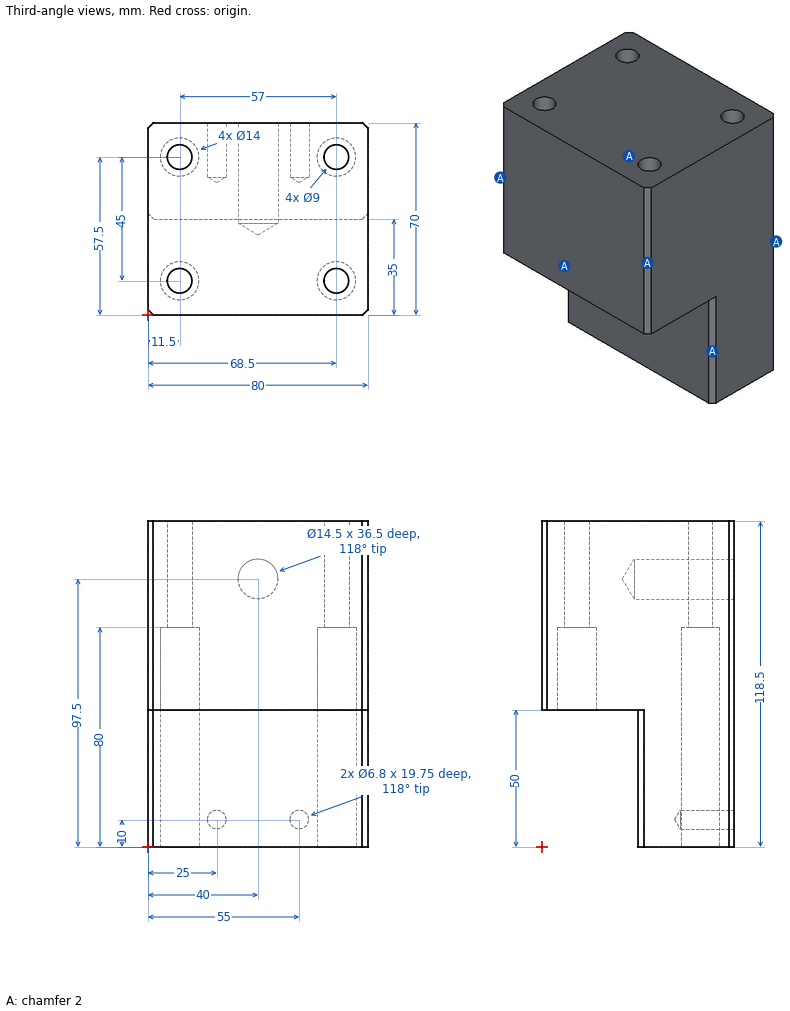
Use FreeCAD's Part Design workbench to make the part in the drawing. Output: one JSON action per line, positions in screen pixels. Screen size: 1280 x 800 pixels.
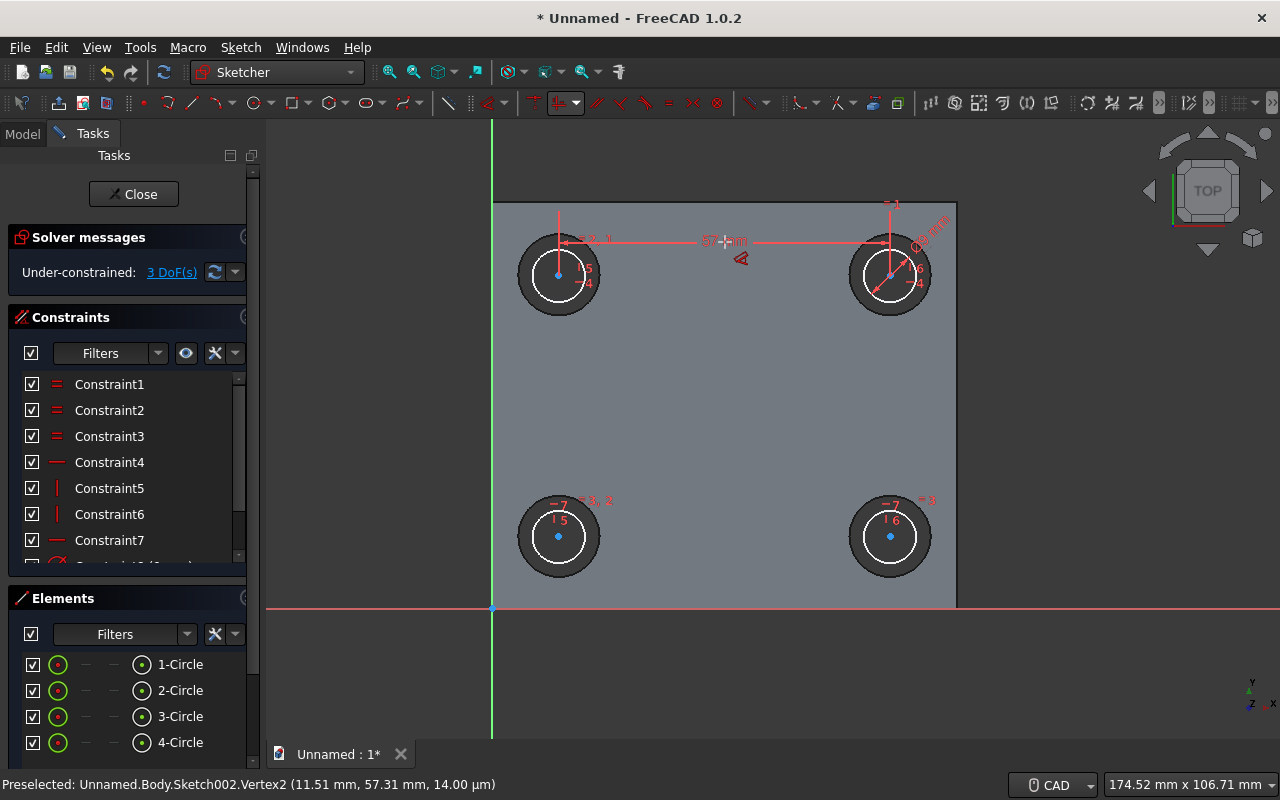
{"action": "left_click", "coordinate": [559, 276]}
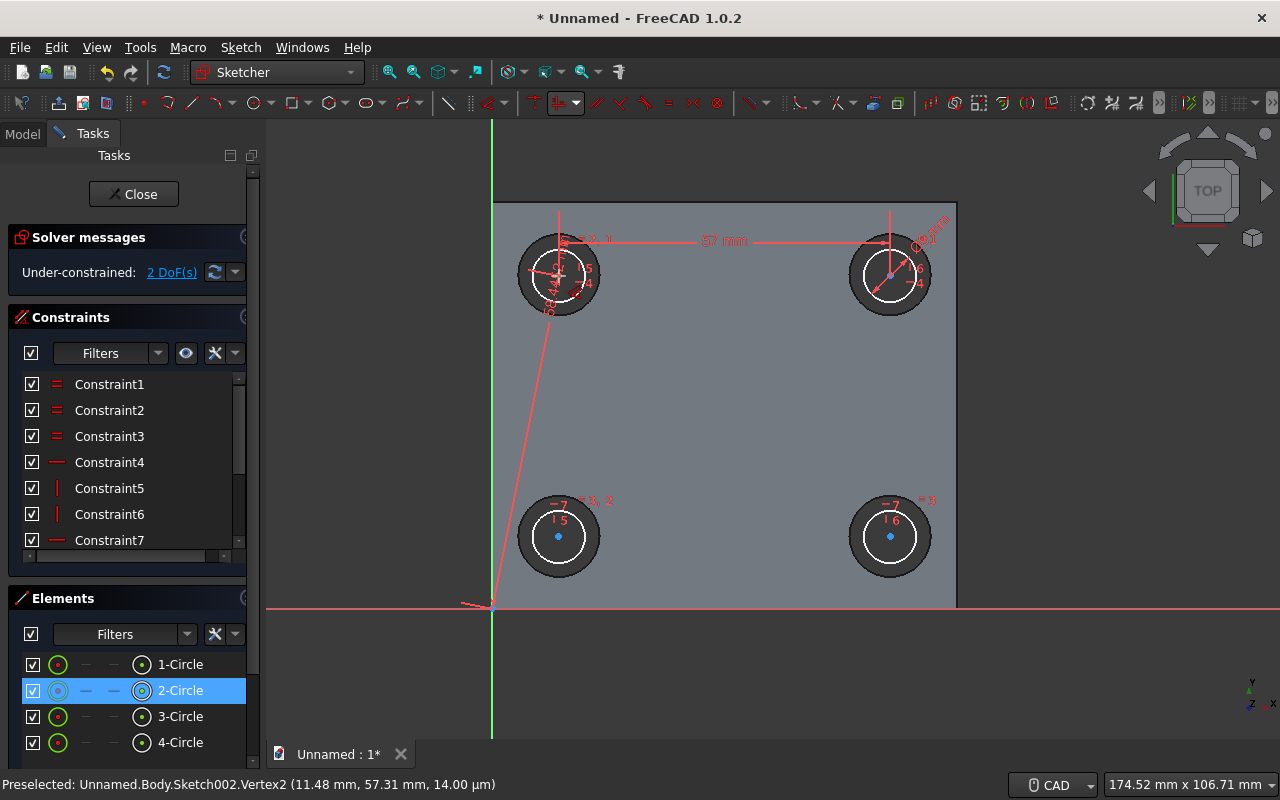
{"action": "left_click", "coordinate": [559, 537]}
{"action": "left_click", "coordinate": [525, 407]}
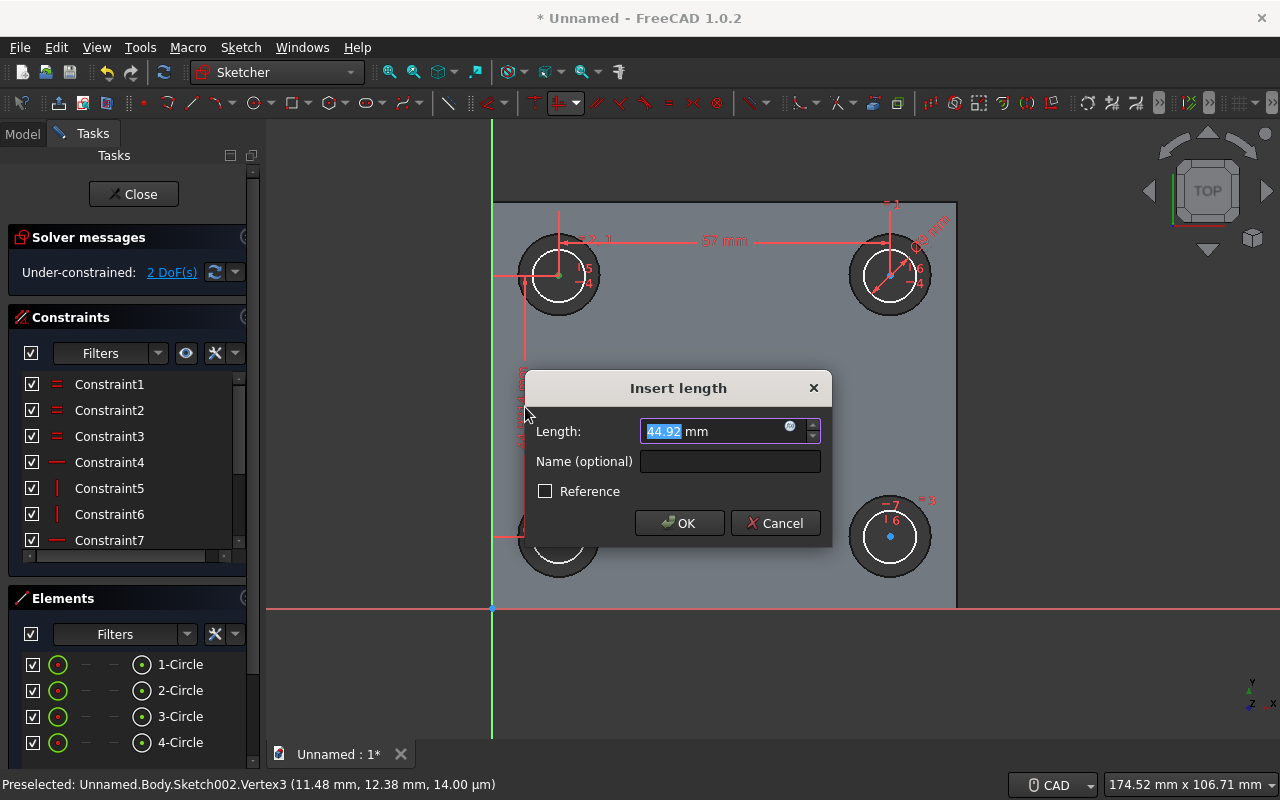
{"action": "type", "text": "45"}
{"action": "key", "text": "Return"}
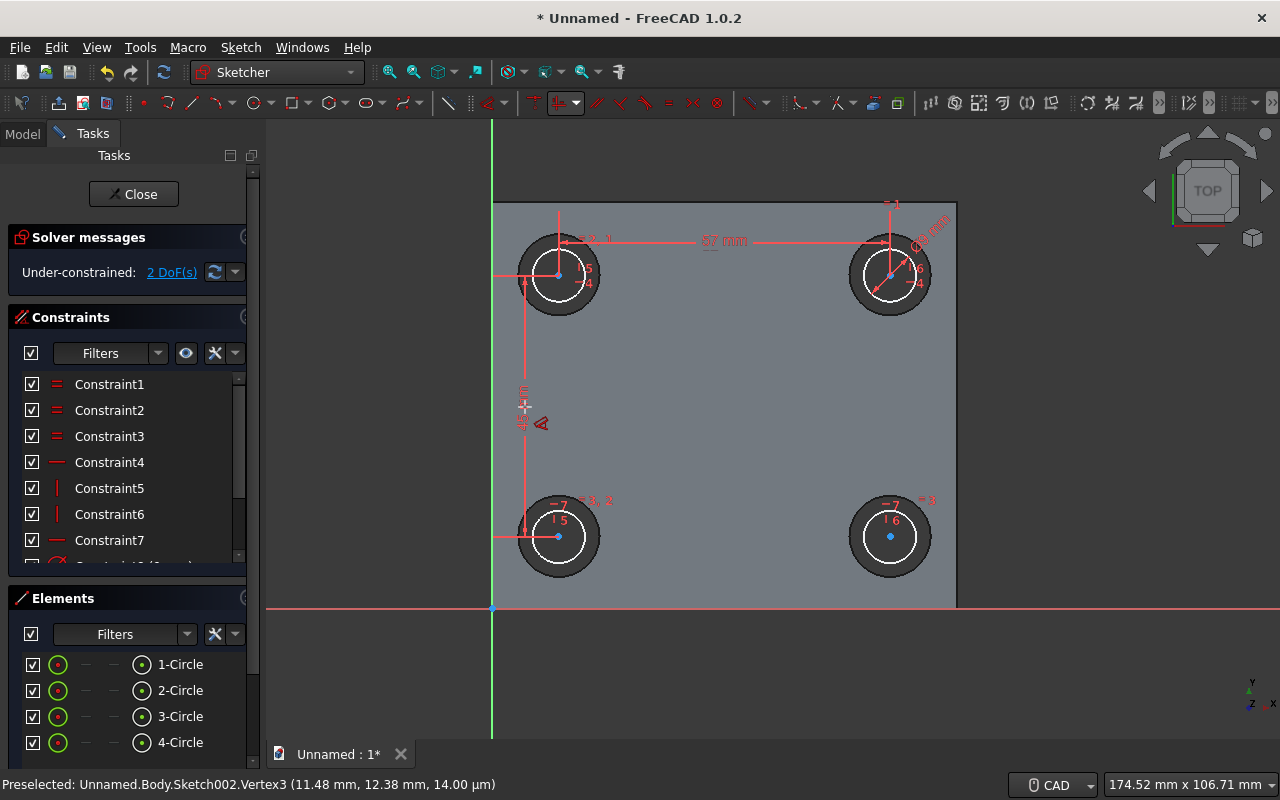
{"action": "left_click", "coordinate": [890, 276]}
{"action": "left_click", "coordinate": [691, 643]}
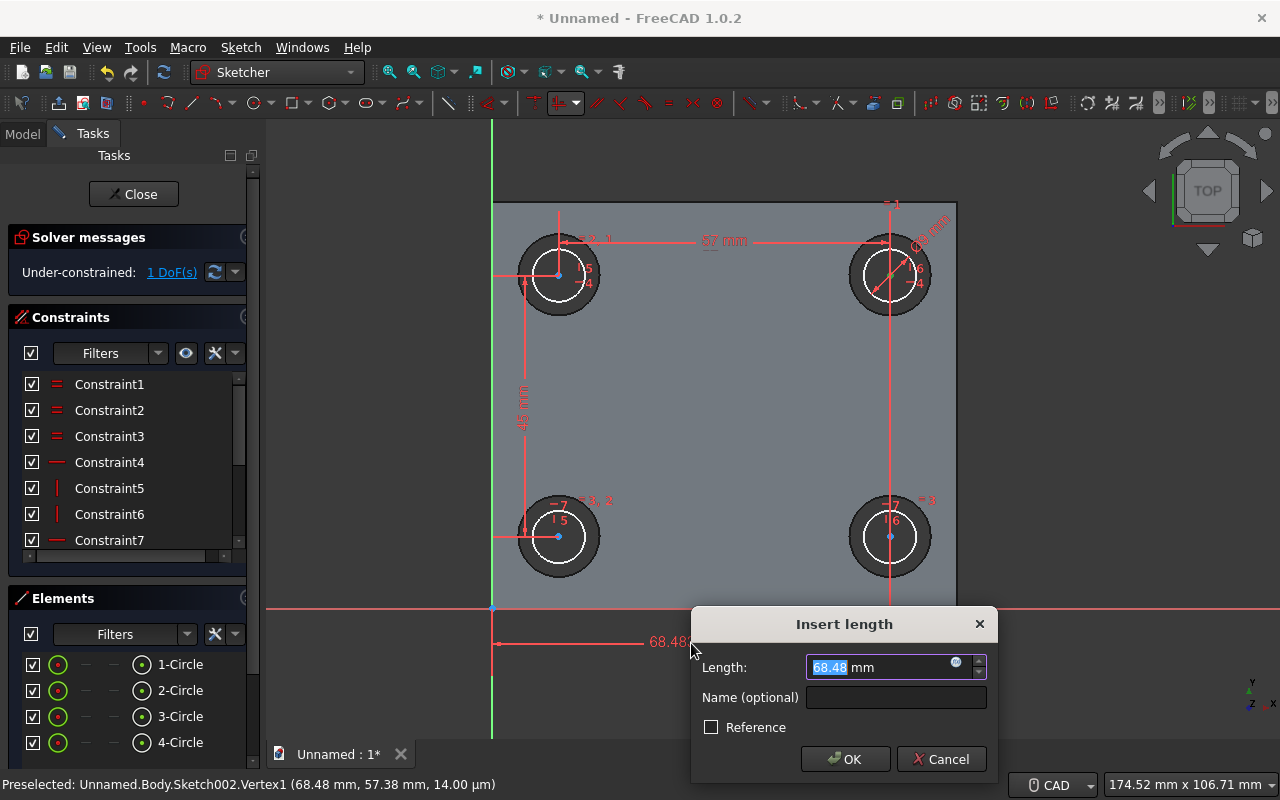
{"action": "type", "text": "68.5"}
{"action": "key", "text": "Return"}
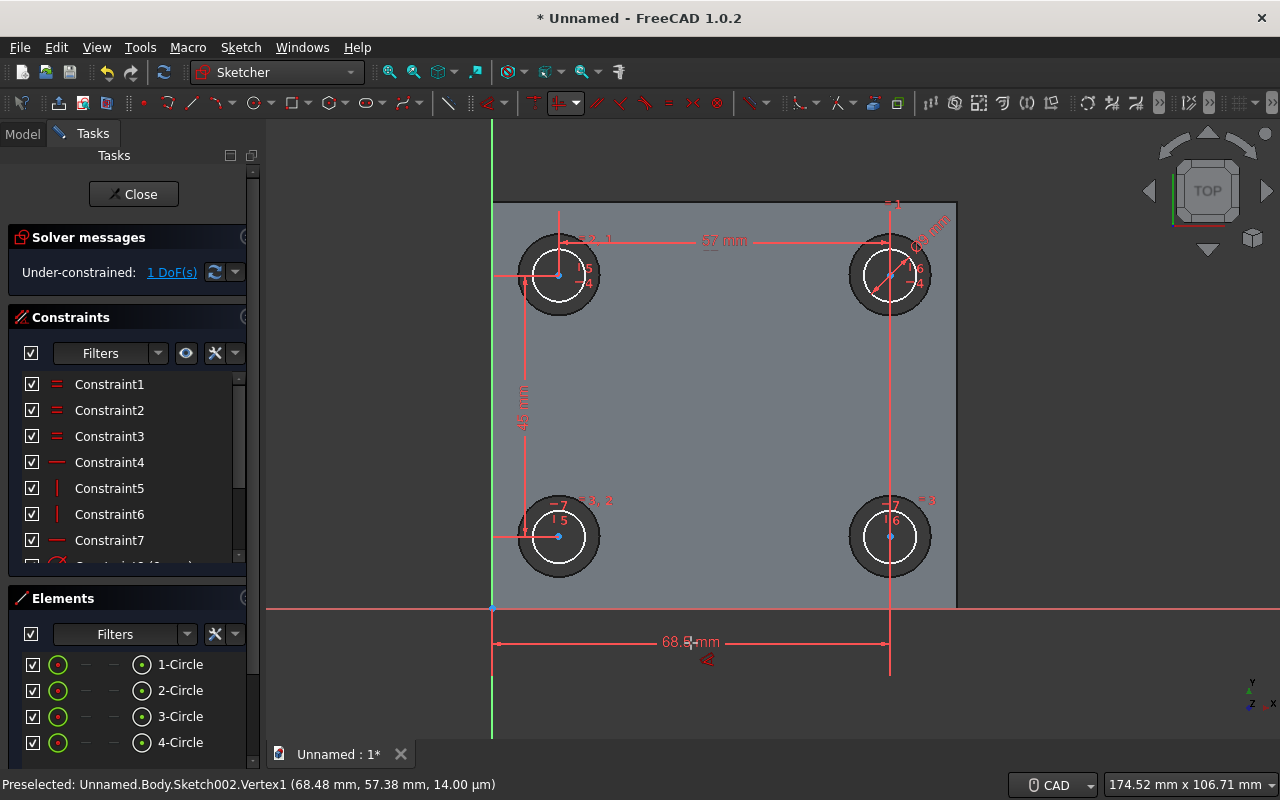
{"action": "left_click", "coordinate": [890, 276]}
{"action": "left_click", "coordinate": [458, 442]}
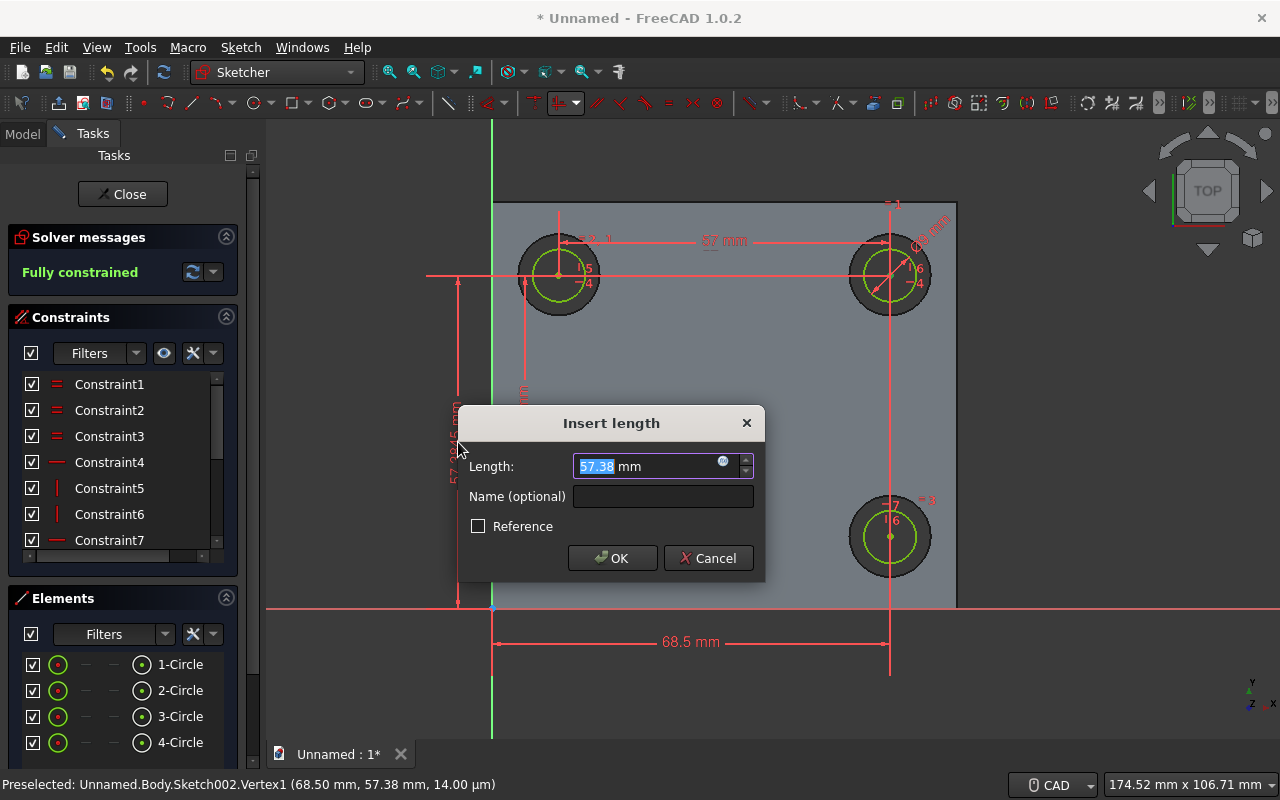
{"action": "type", "text": "57.5"}
{"action": "key", "text": "Return"}
{"action": "key", "text": "Escape"}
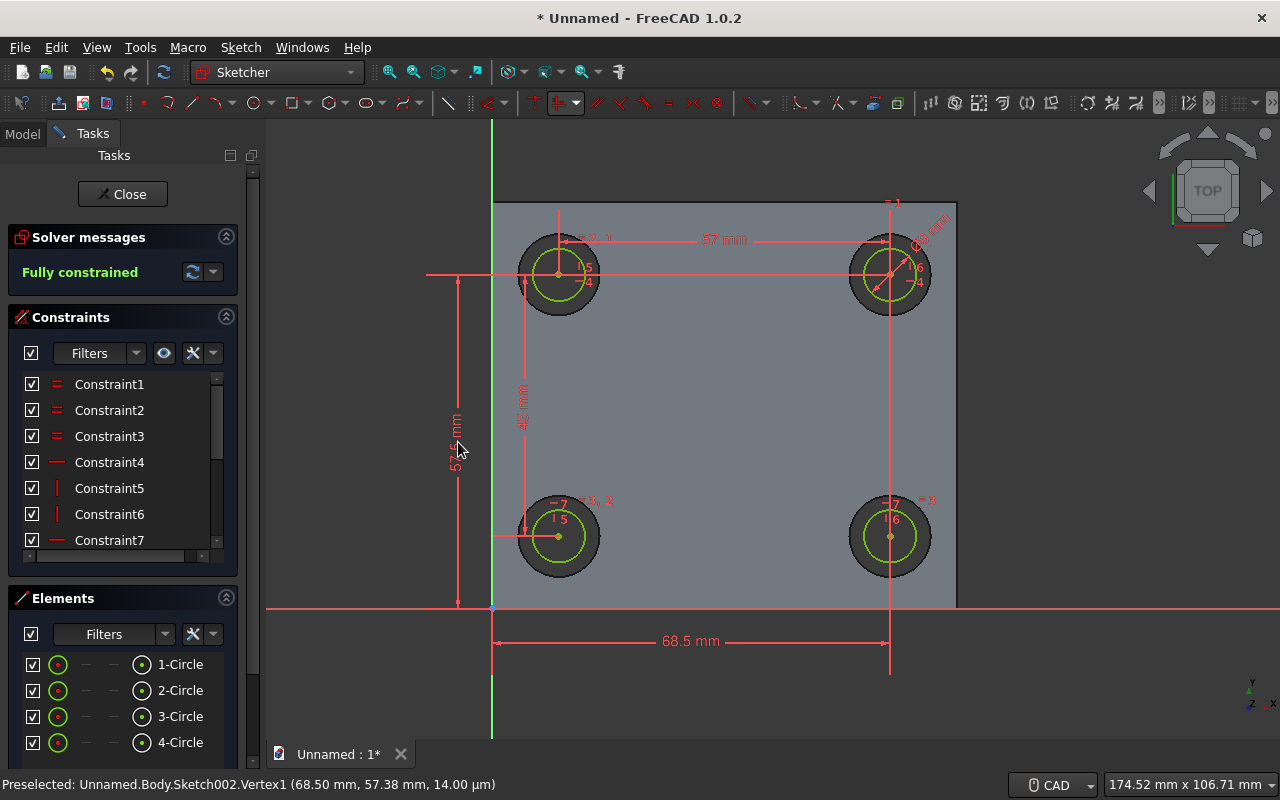
{"action": "left_click", "coordinate": [123, 194]}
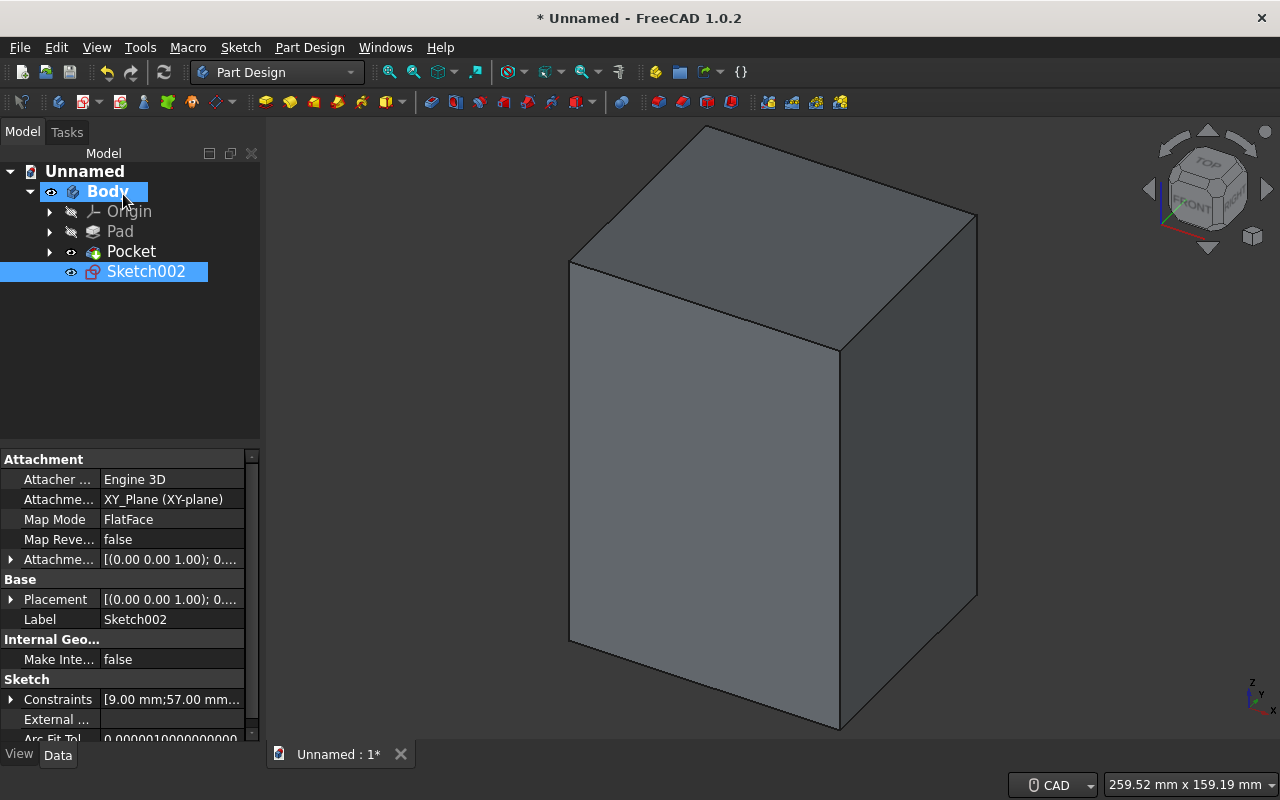
{"action": "left_click", "coordinate": [432, 102]}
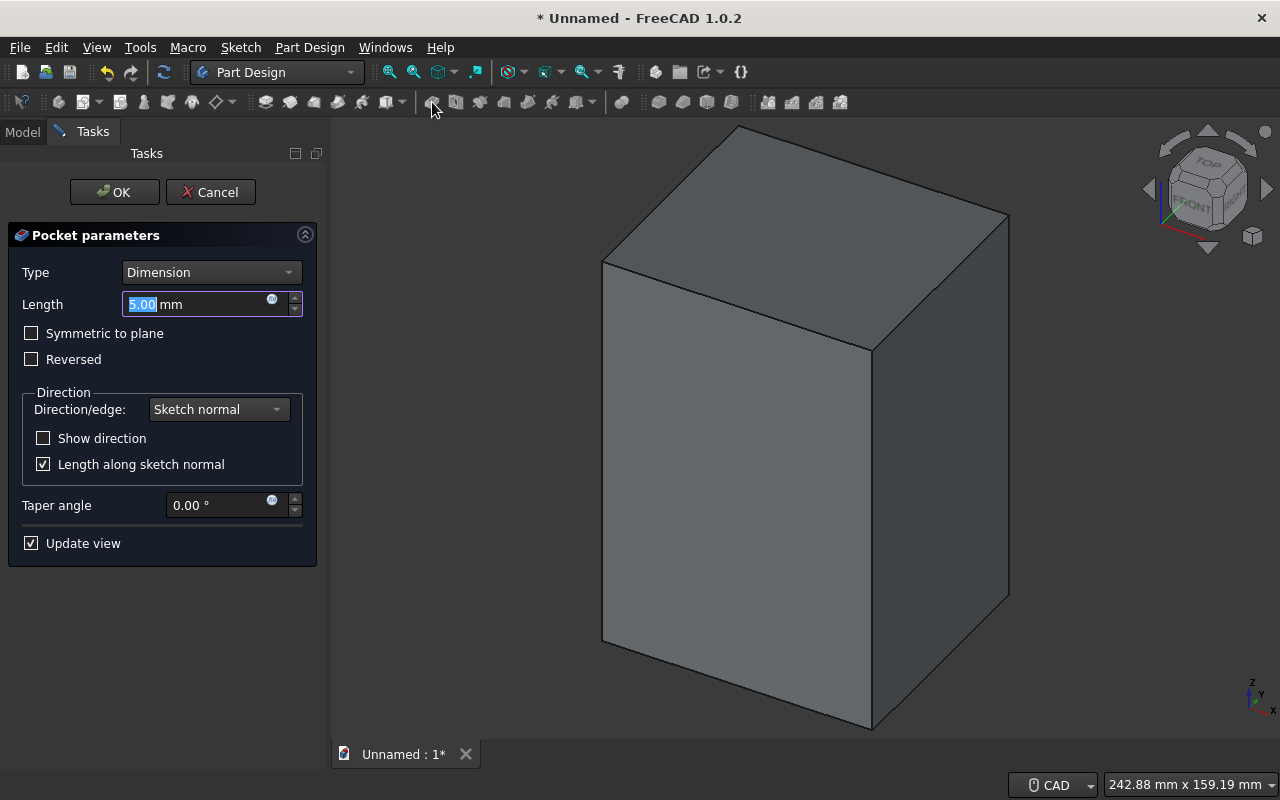
{"action": "left_click", "coordinate": [212, 272]}